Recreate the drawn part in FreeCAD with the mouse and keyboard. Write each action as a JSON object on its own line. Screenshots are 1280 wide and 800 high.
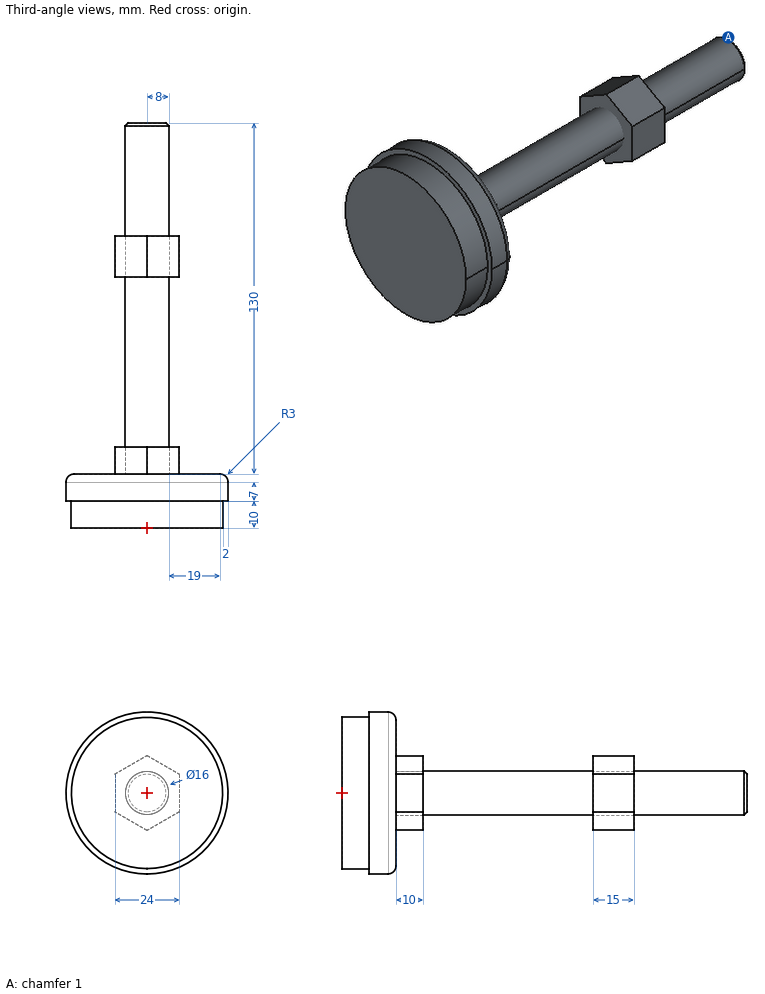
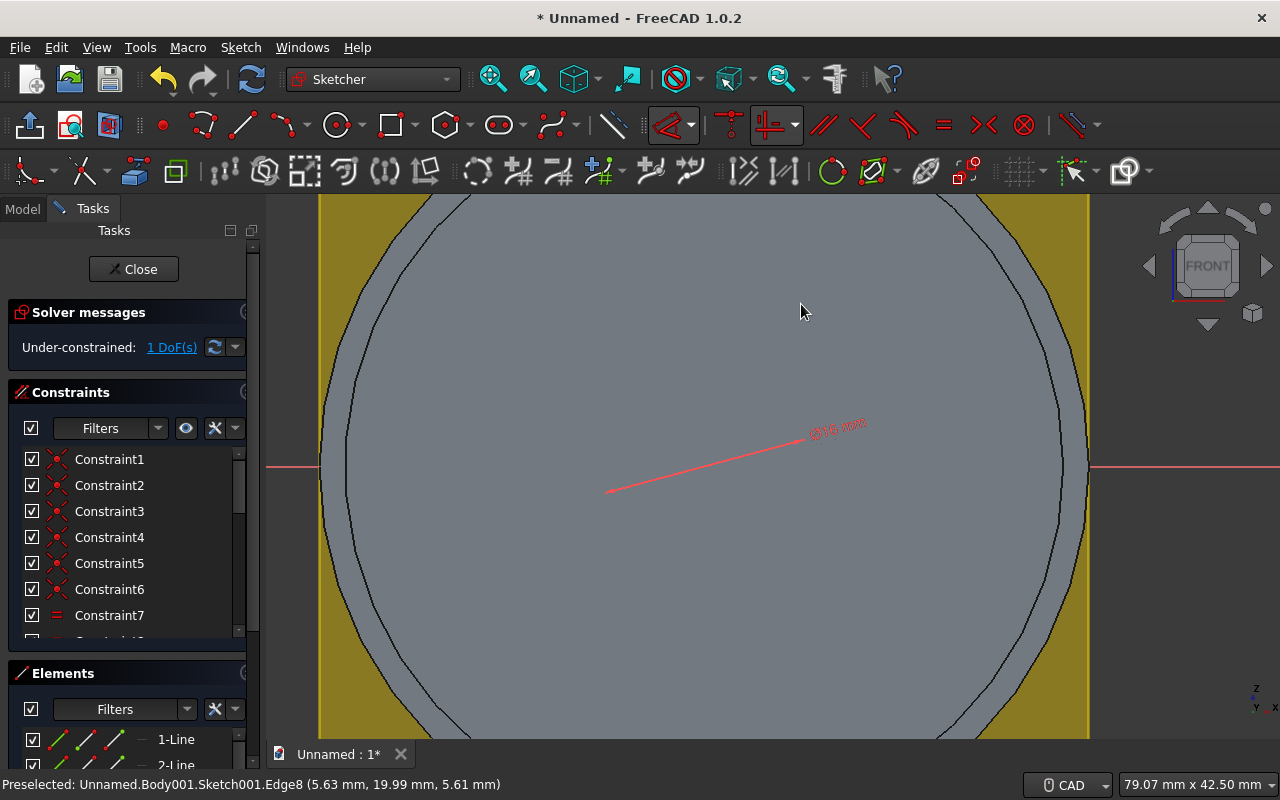
{"action": "left_click", "coordinate": [550, 377]}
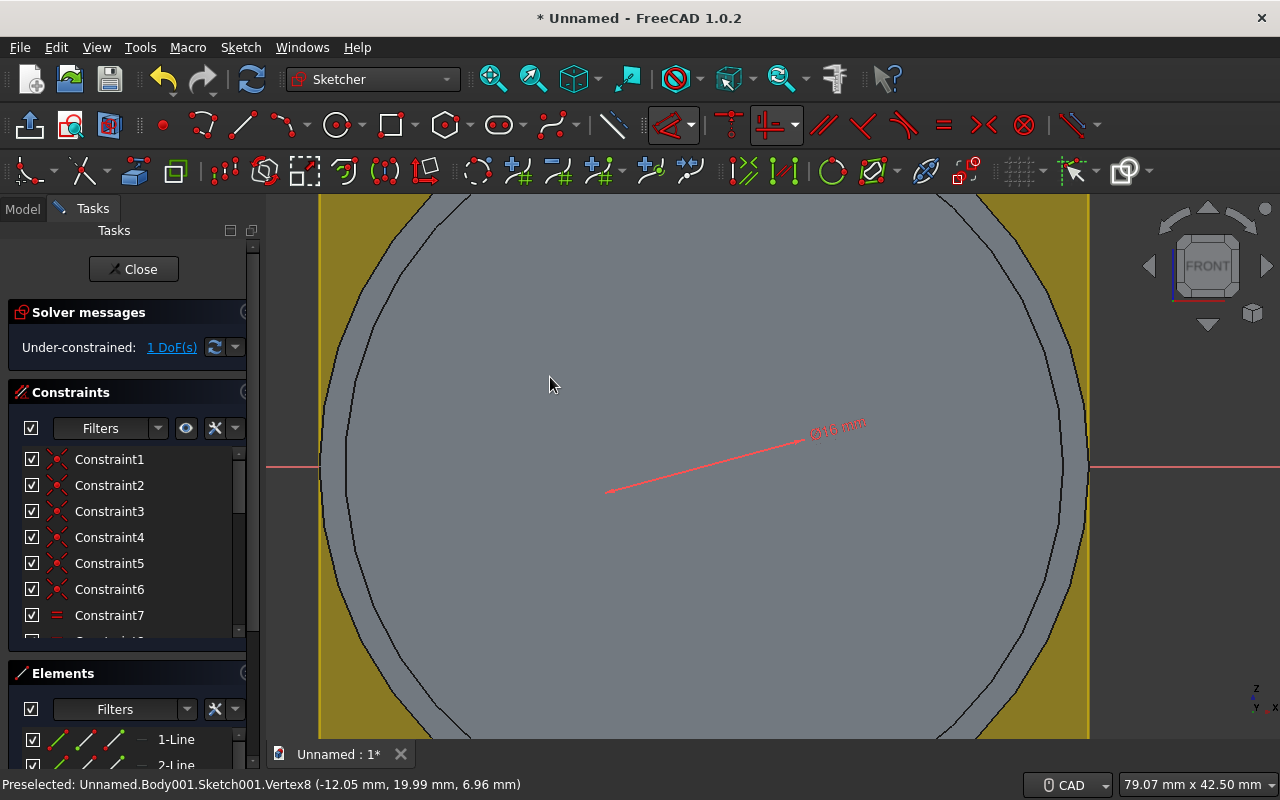
{"action": "left_click", "coordinate": [859, 556]}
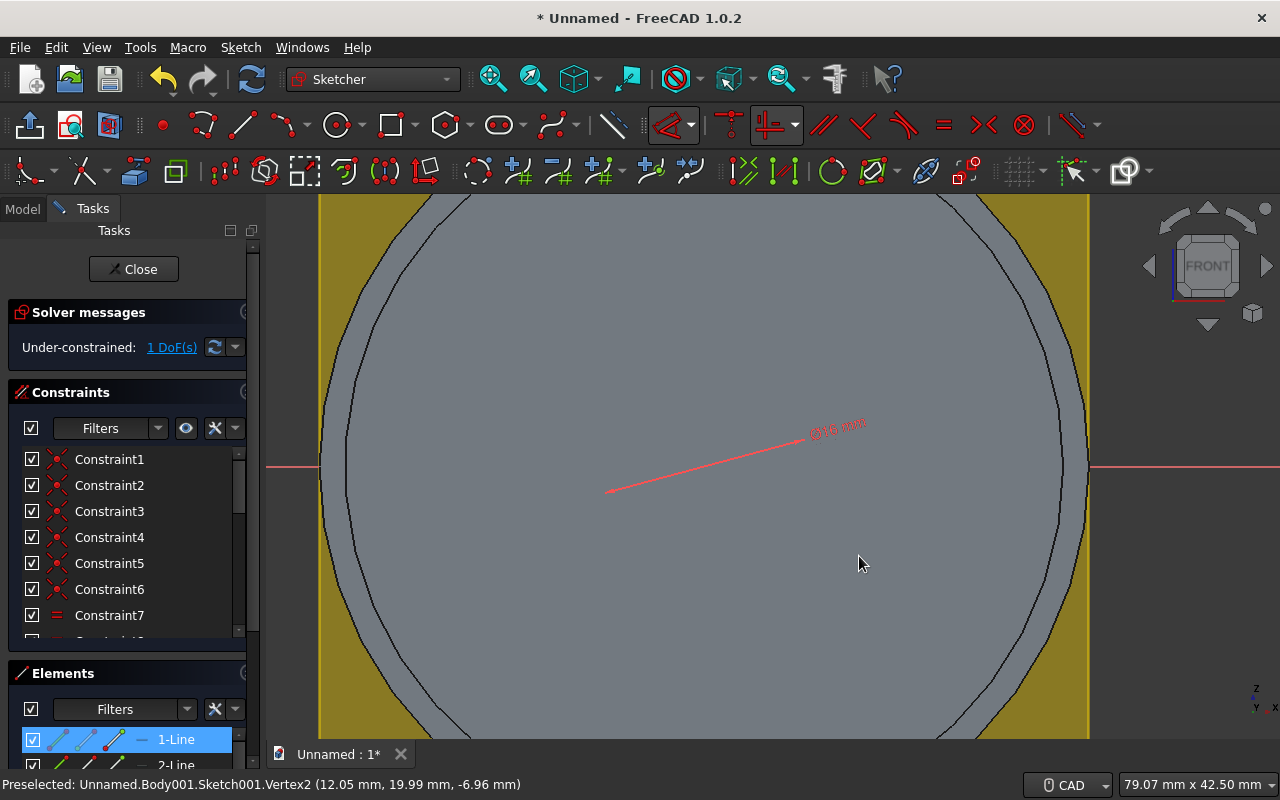
{"action": "key", "text": "l"}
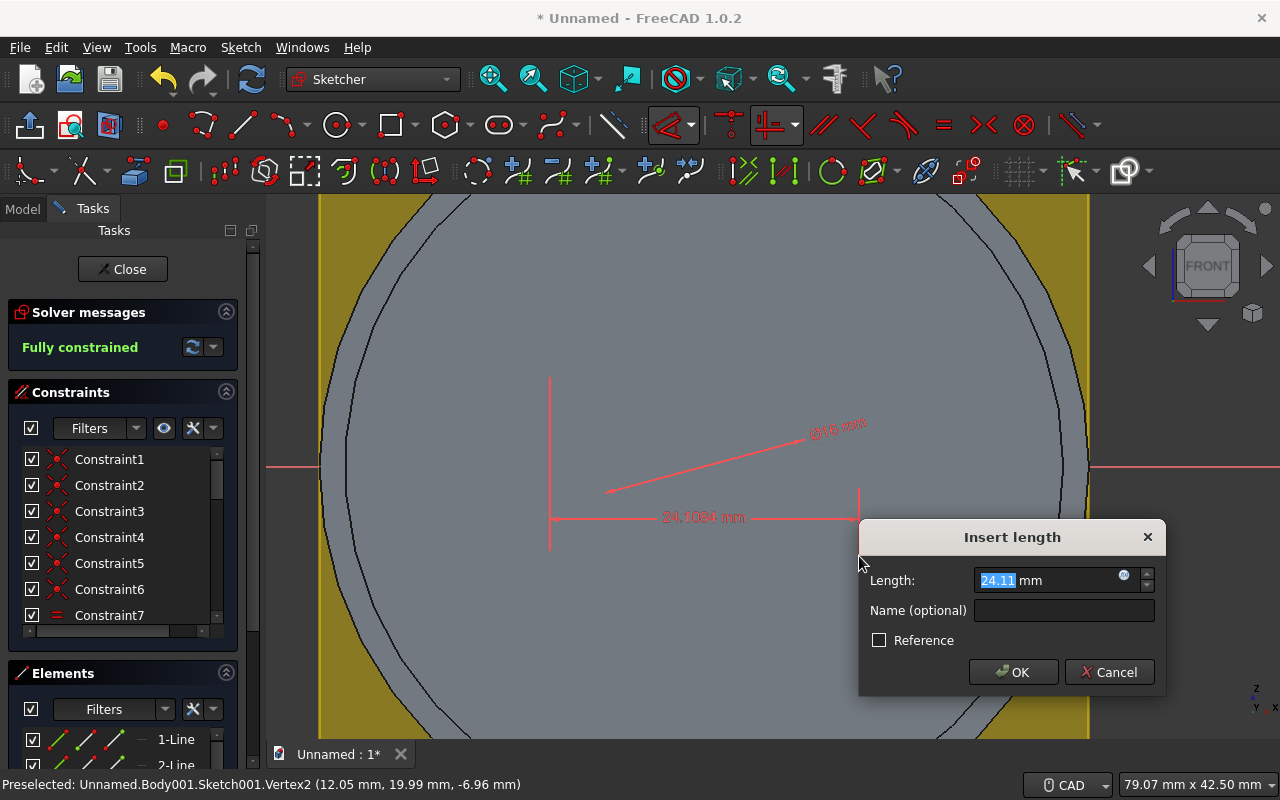
{"action": "type", "text": "24"}
{"action": "key", "text": "Return"}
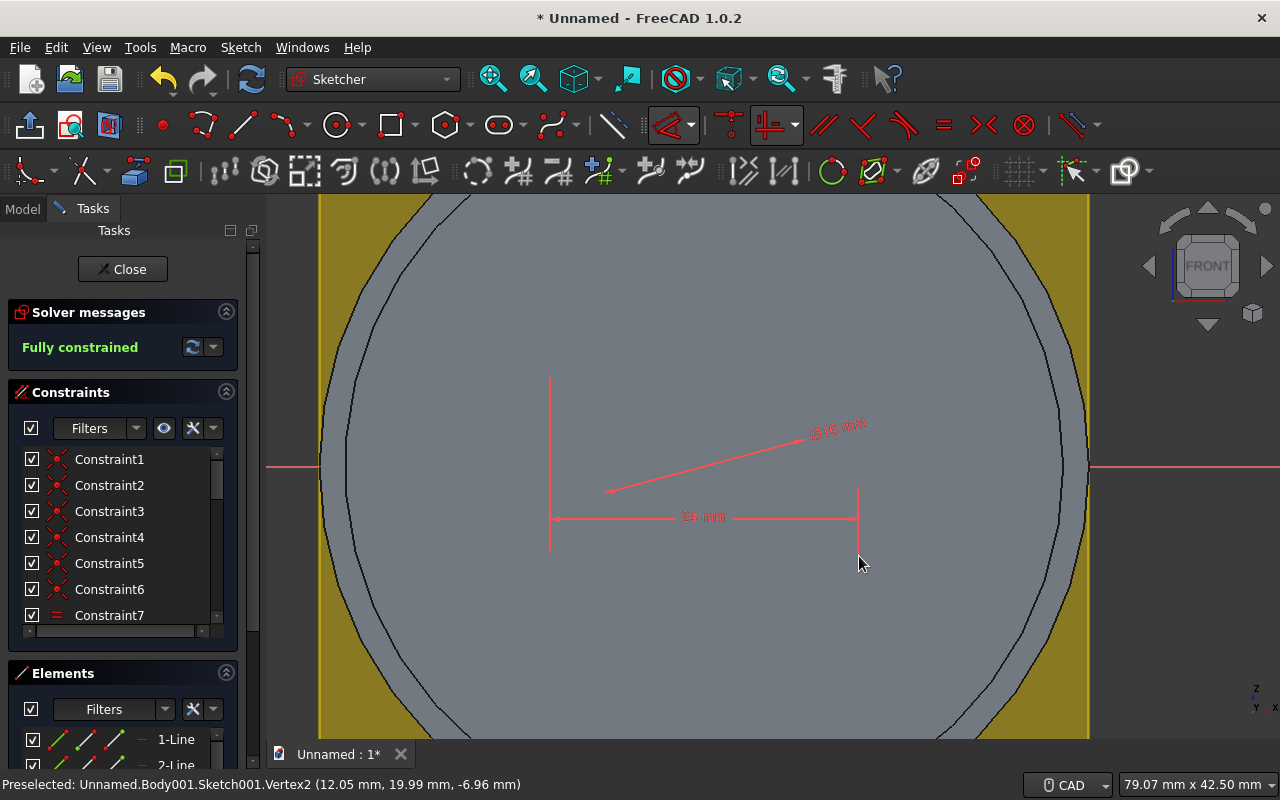
{"action": "left_click", "coordinate": [123, 269]}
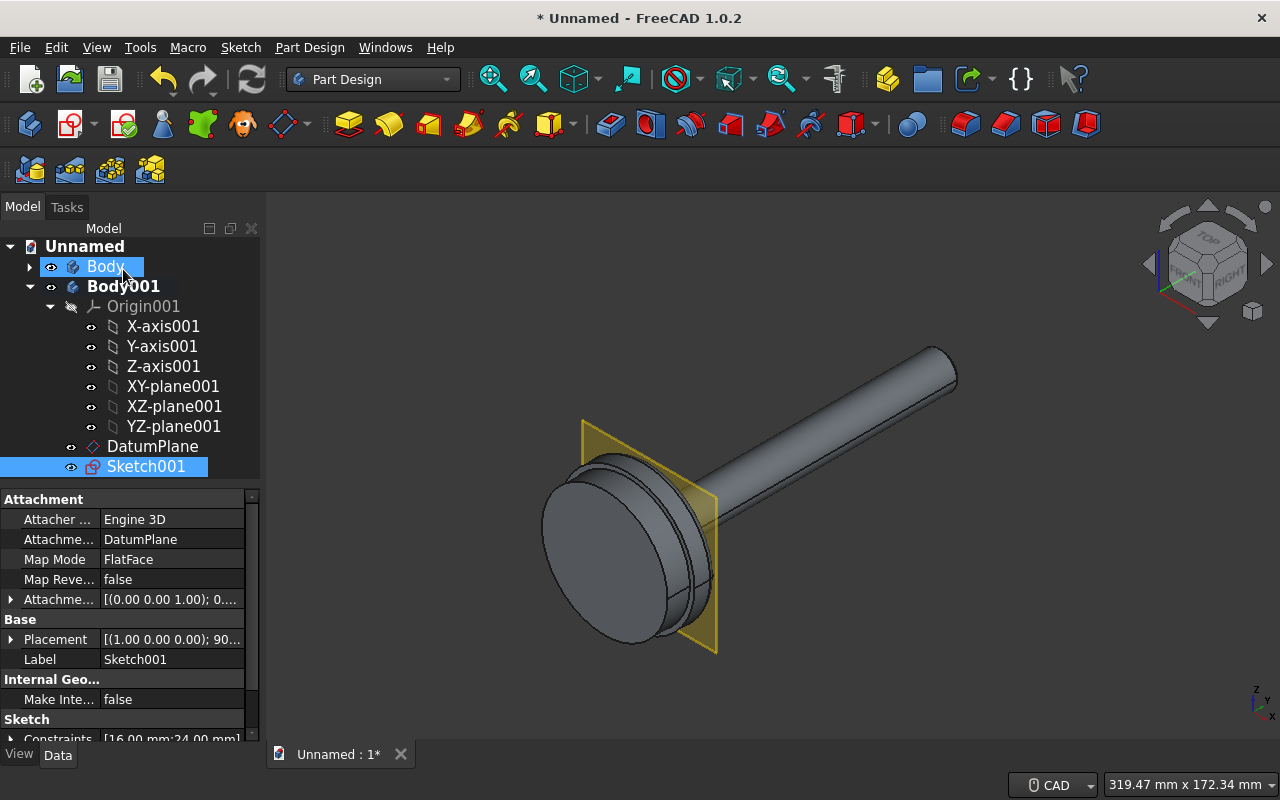
{"action": "left_click", "coordinate": [350, 124]}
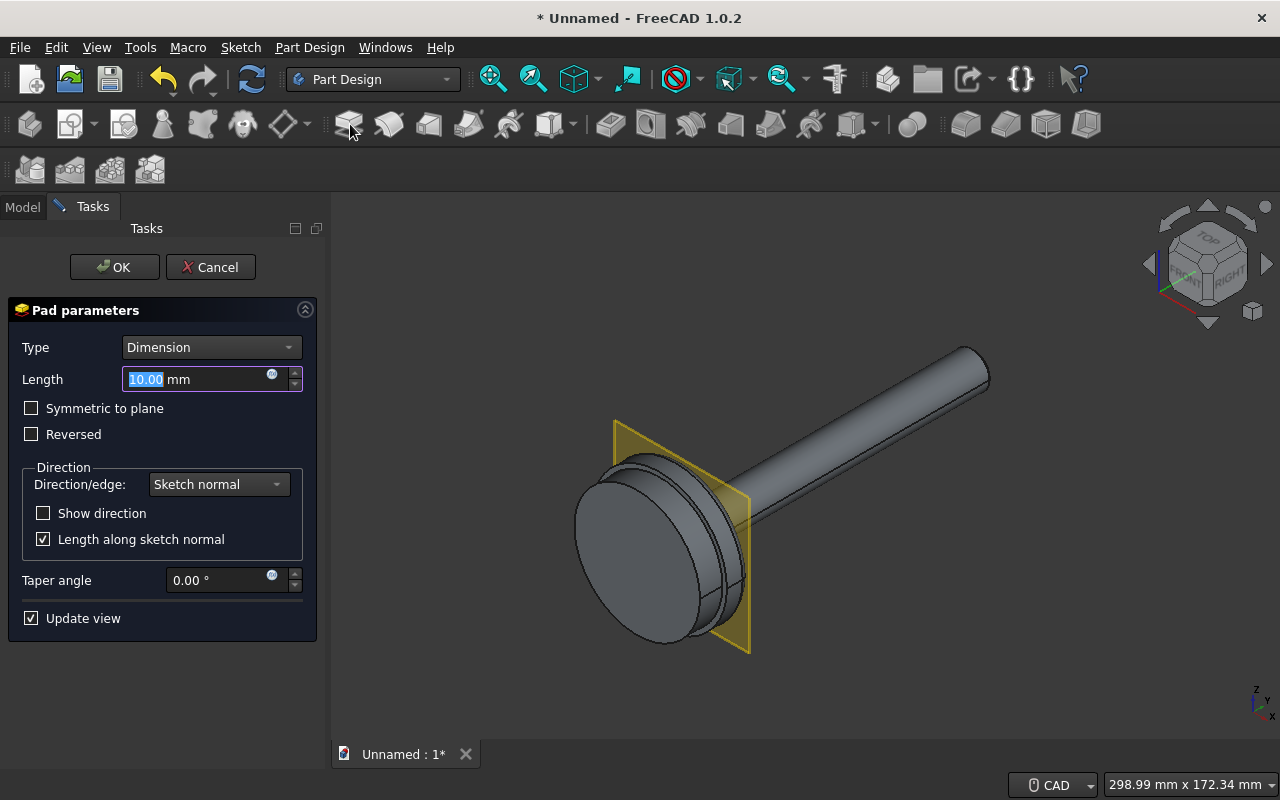
{"action": "type", "text": "10"}
{"action": "key", "text": "Tab"}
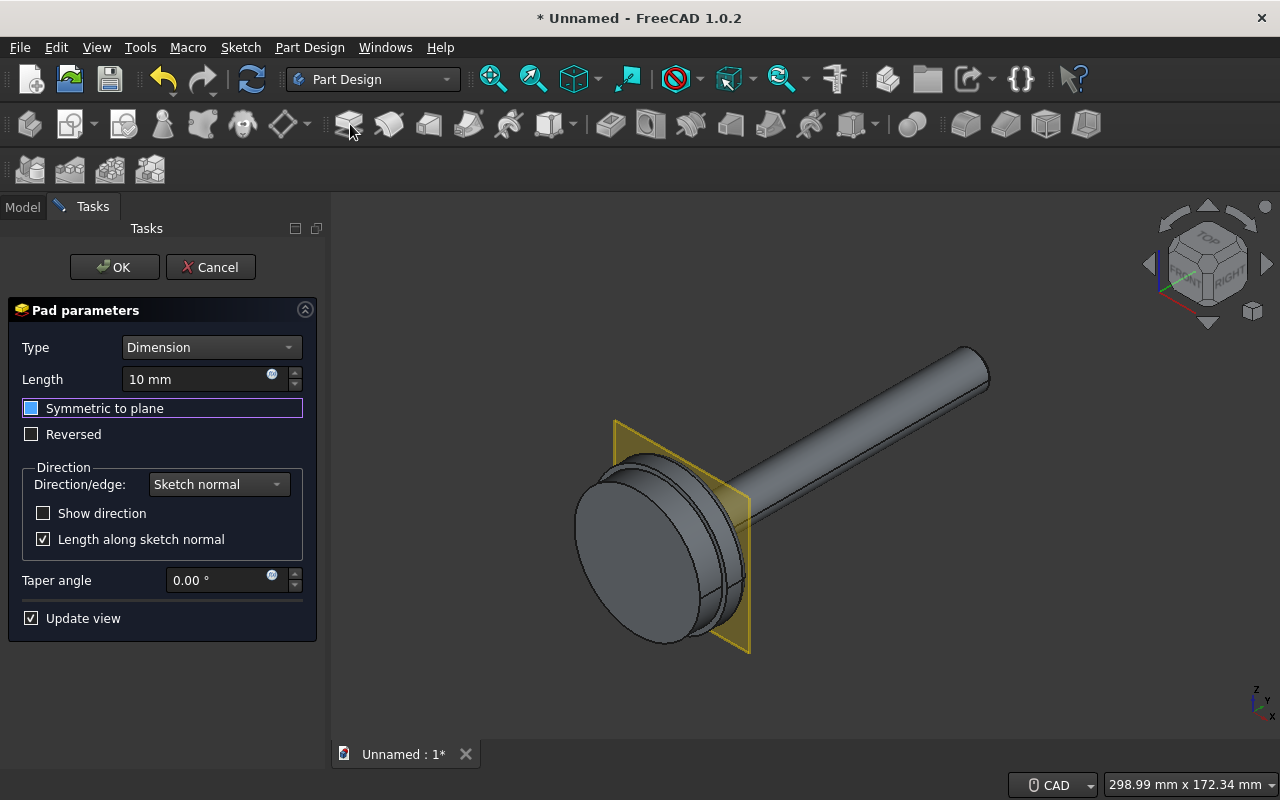
{"action": "left_click", "coordinate": [30, 434]}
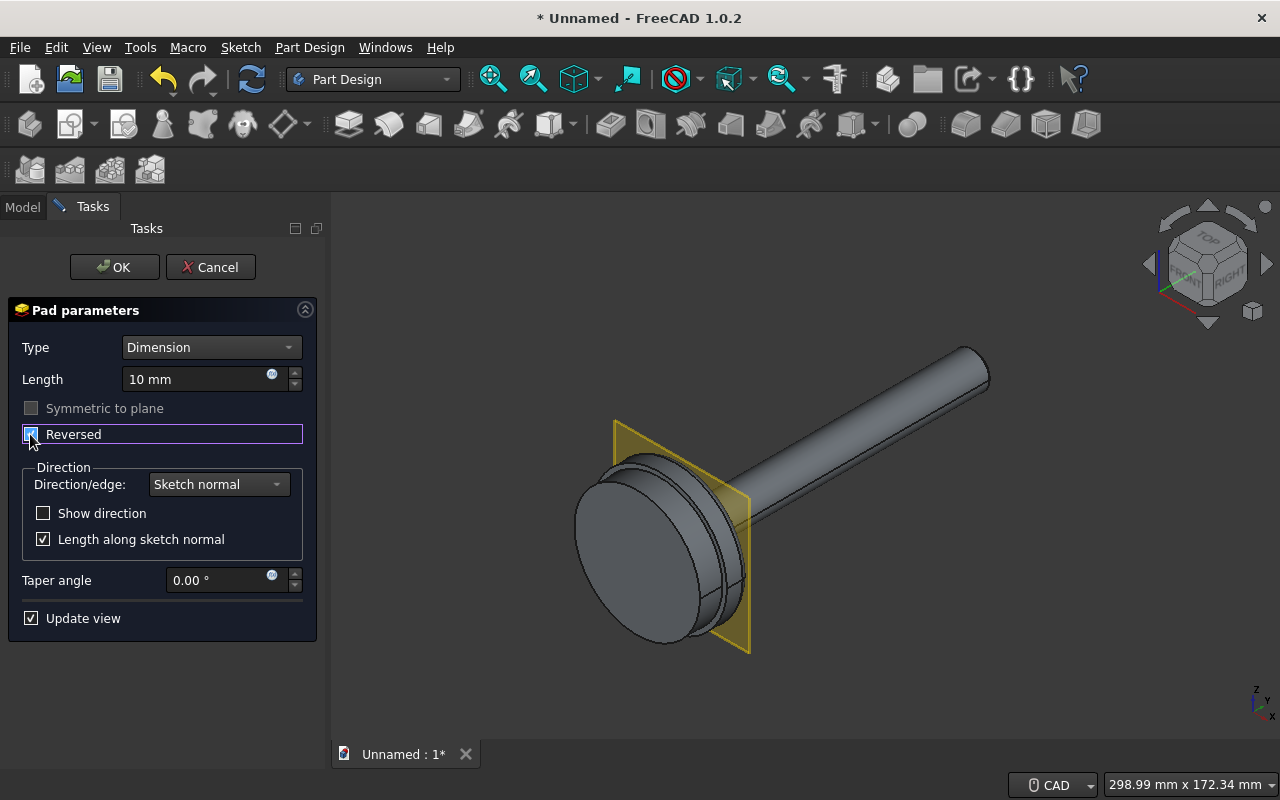
{"action": "left_click", "coordinate": [115, 267]}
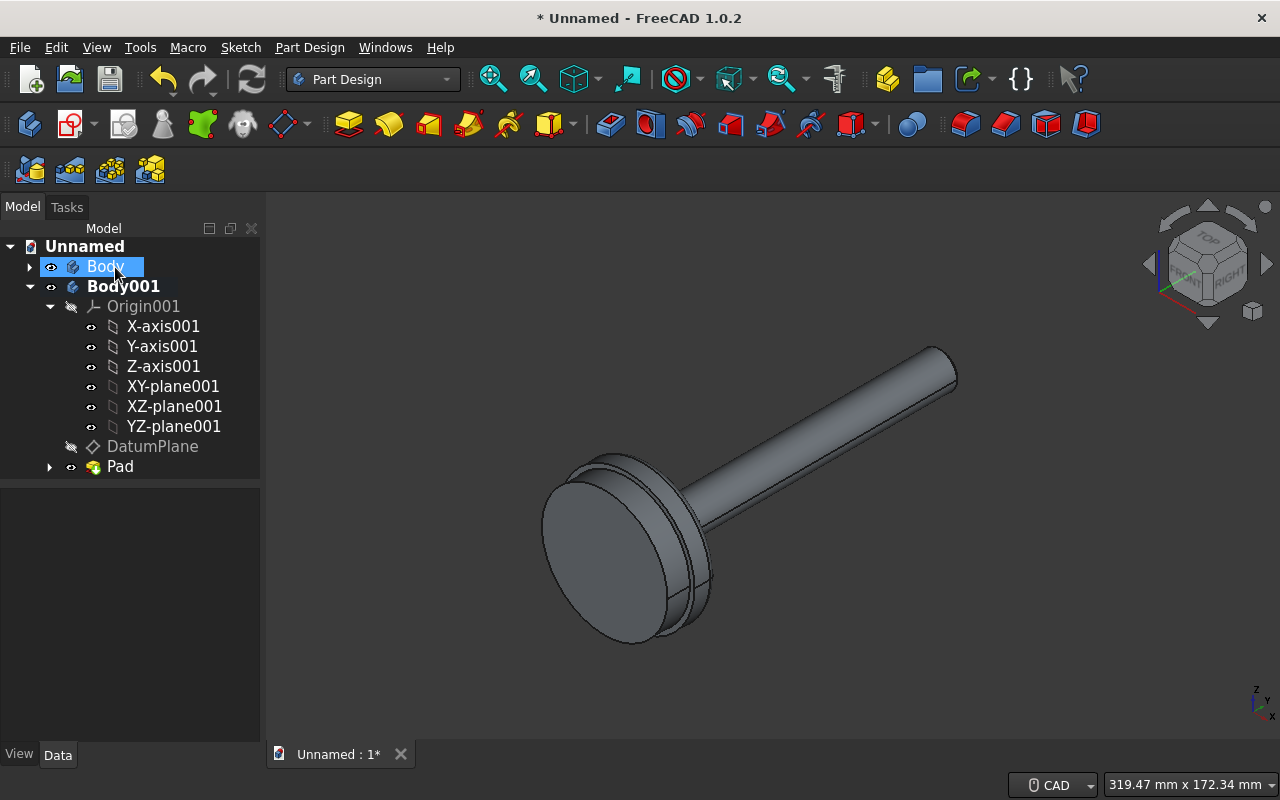
{"action": "left_click", "coordinate": [494, 80]}